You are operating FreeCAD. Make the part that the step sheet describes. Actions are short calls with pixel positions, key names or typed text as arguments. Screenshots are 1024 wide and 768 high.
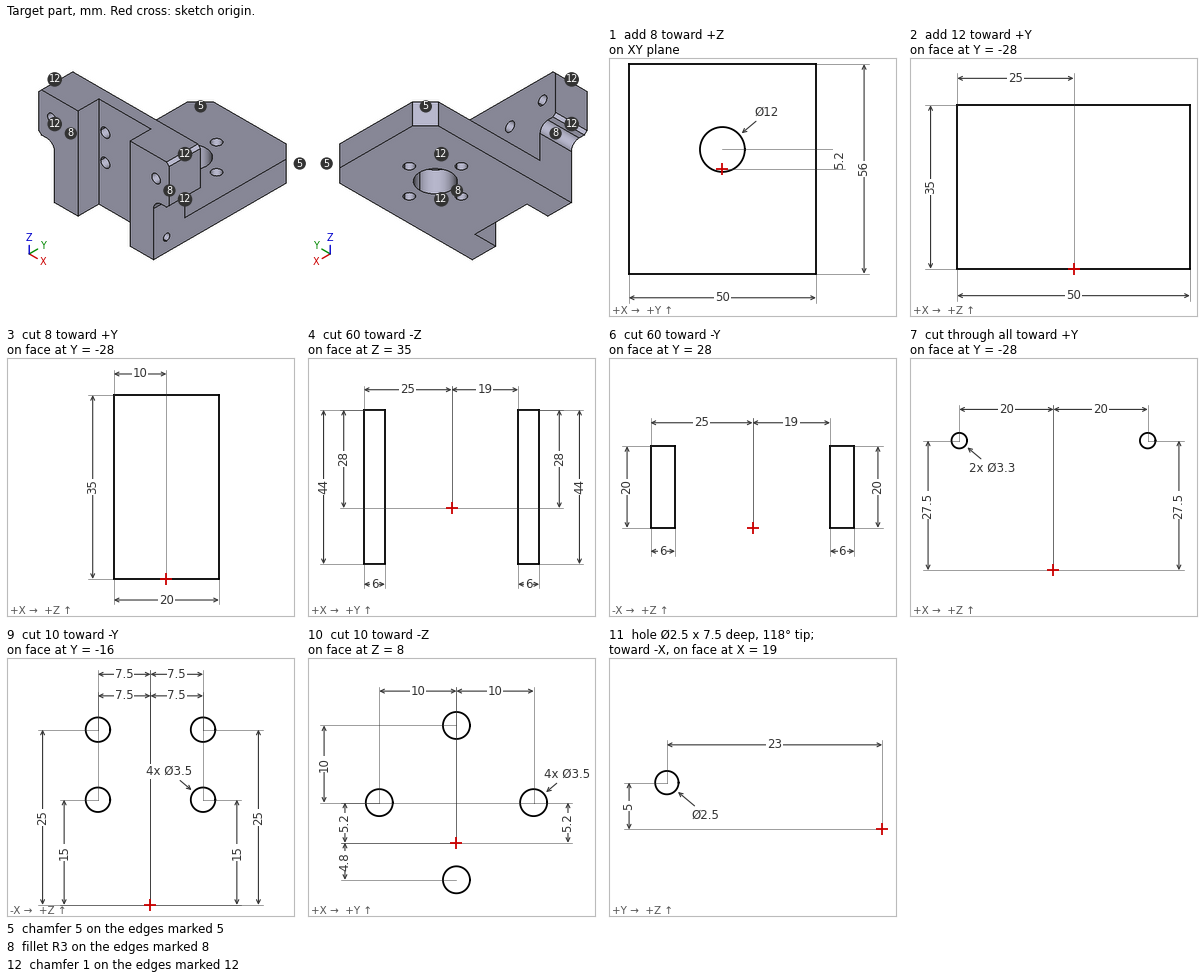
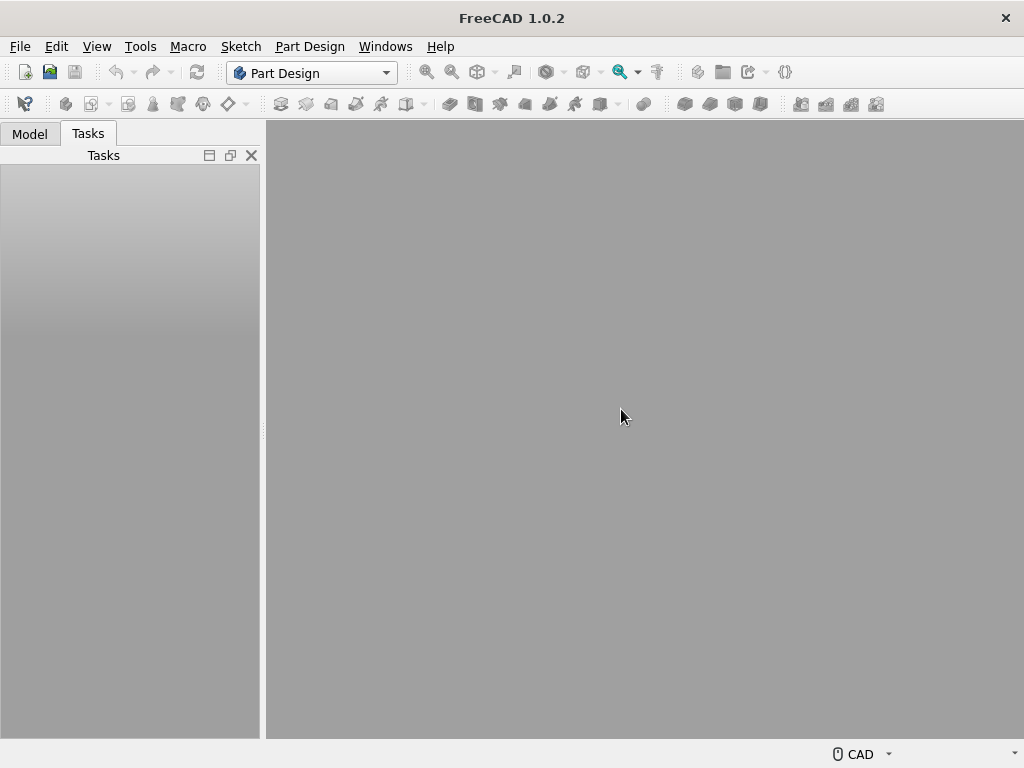
click(25, 72)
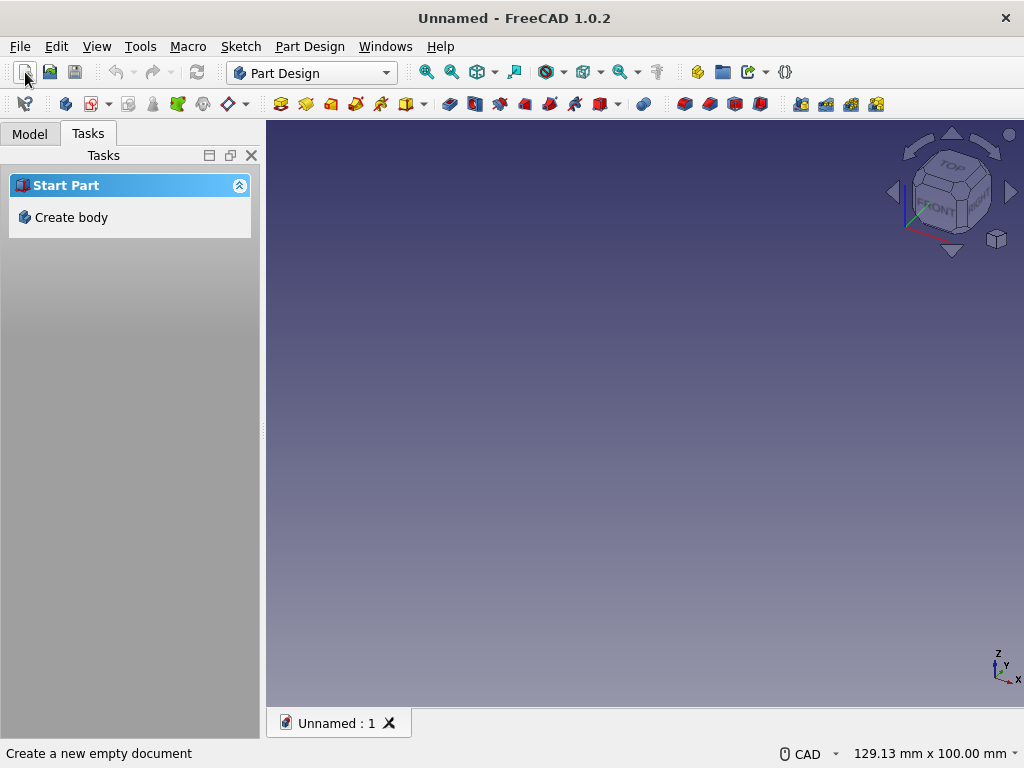
click(90, 104)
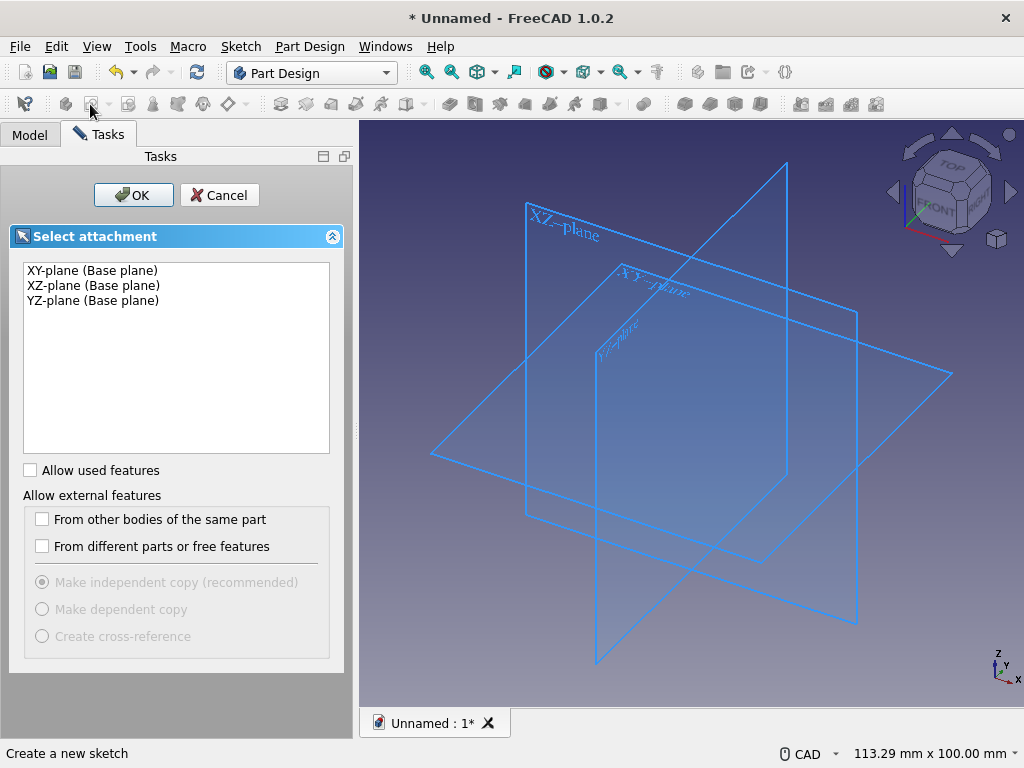
click(84, 270)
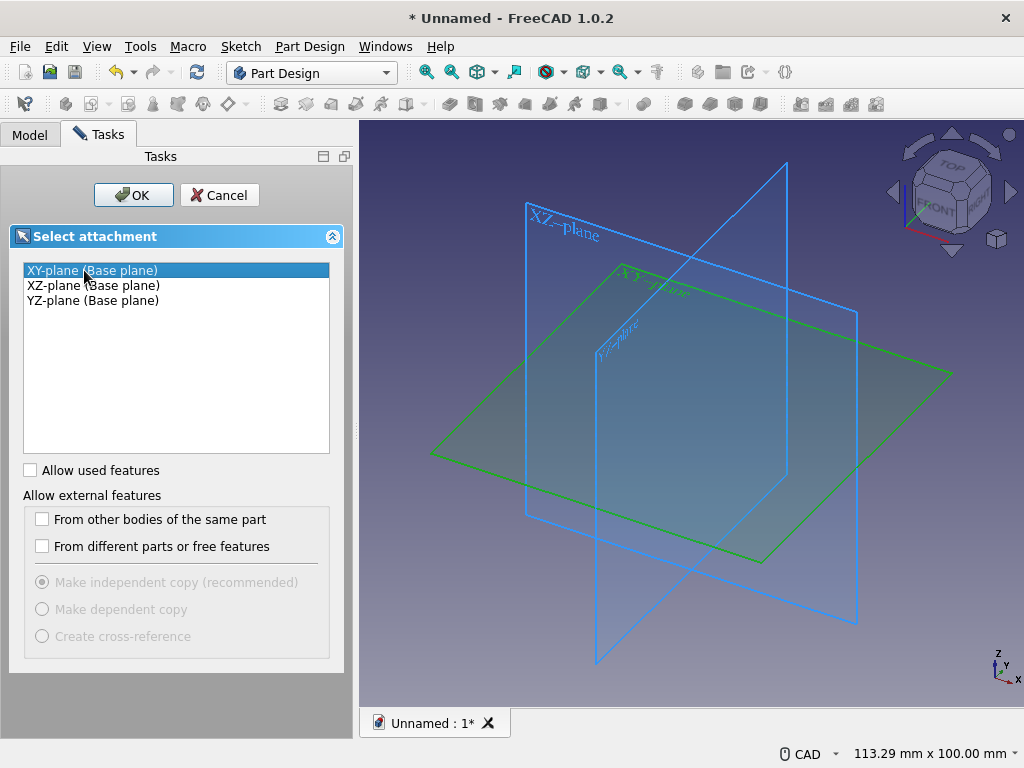
click(134, 195)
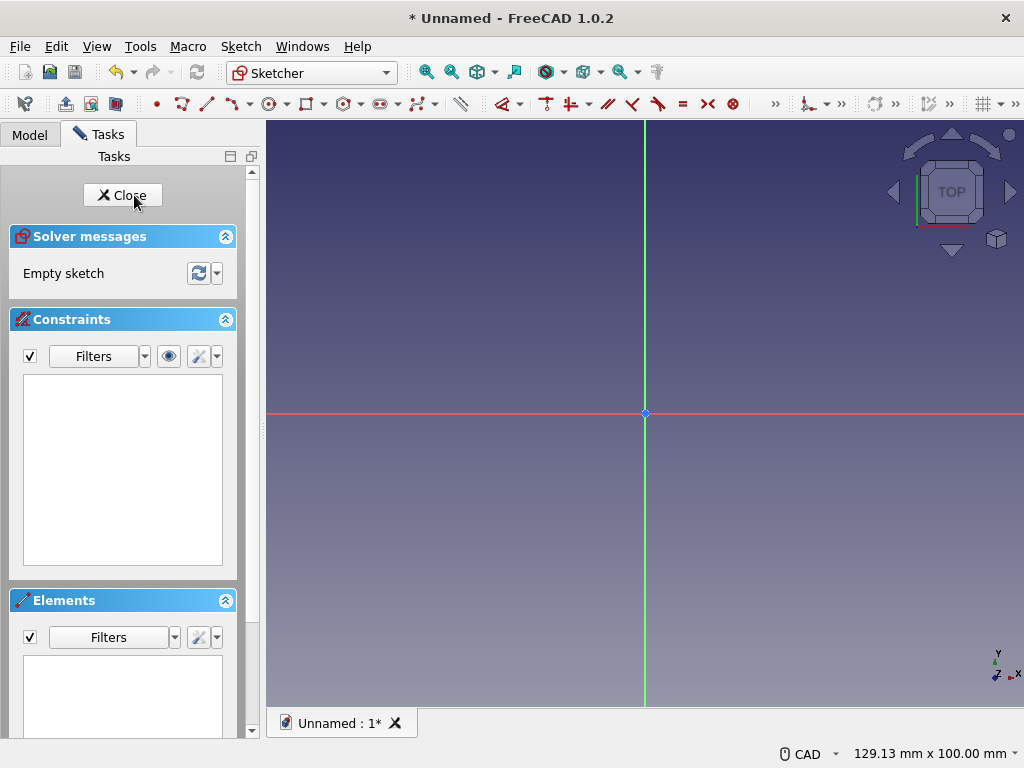
key(g)
key(v)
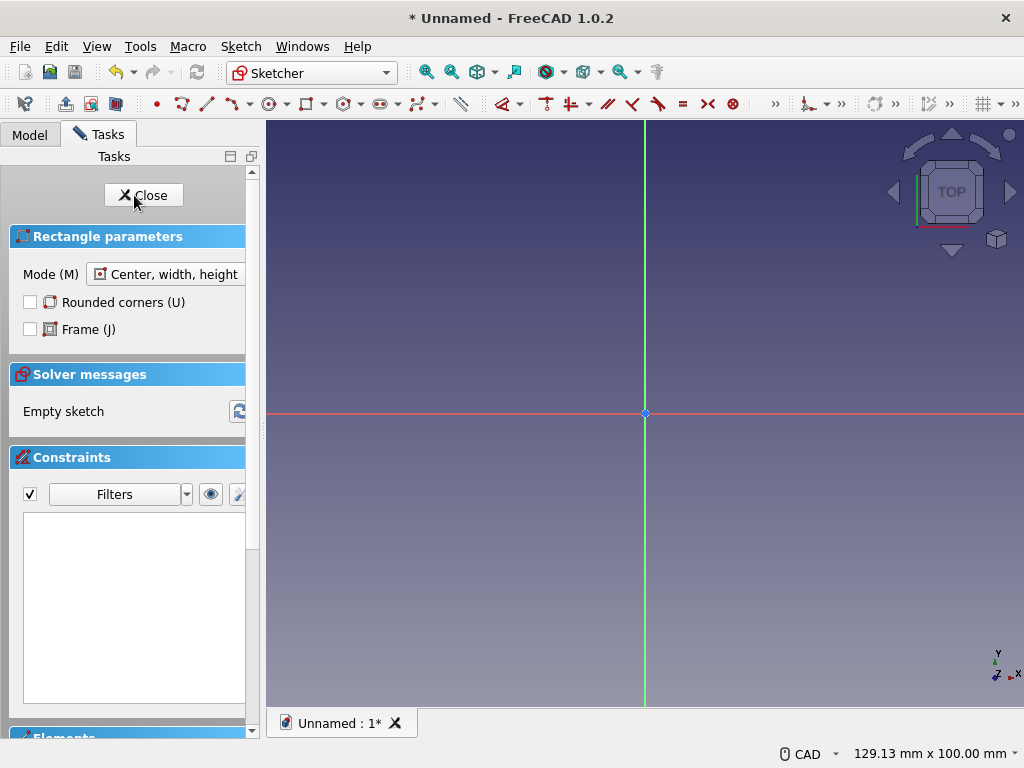
click(645, 414)
move(792, 249)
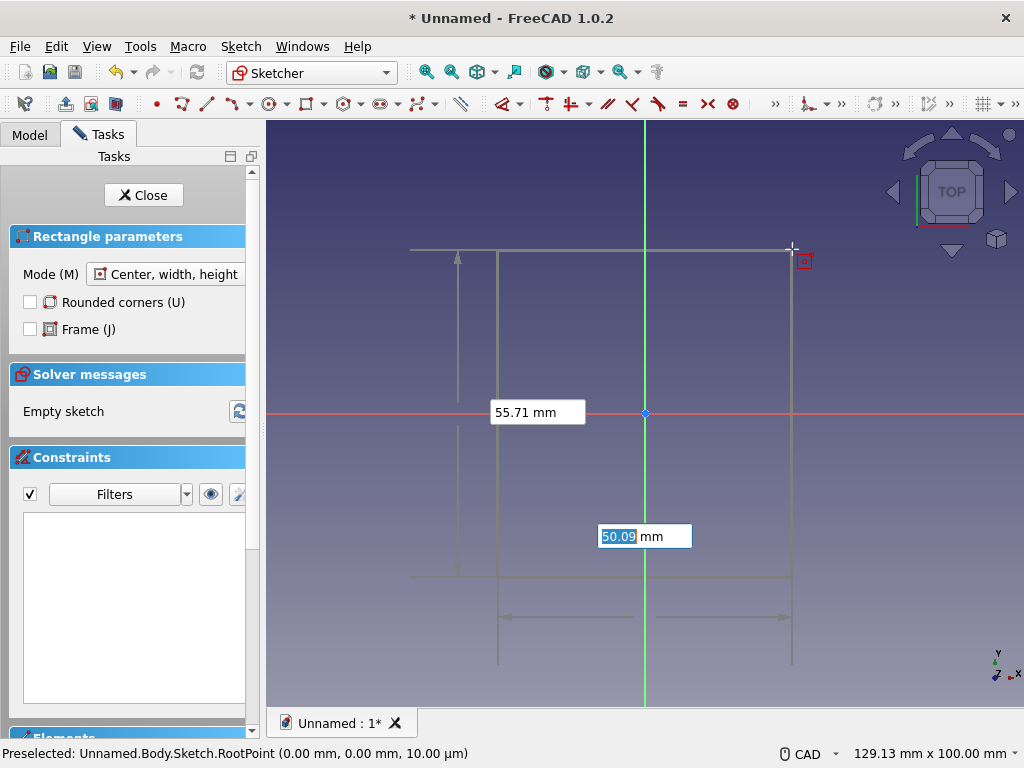
text(50)
key(Tab)
text(56)
key(Return)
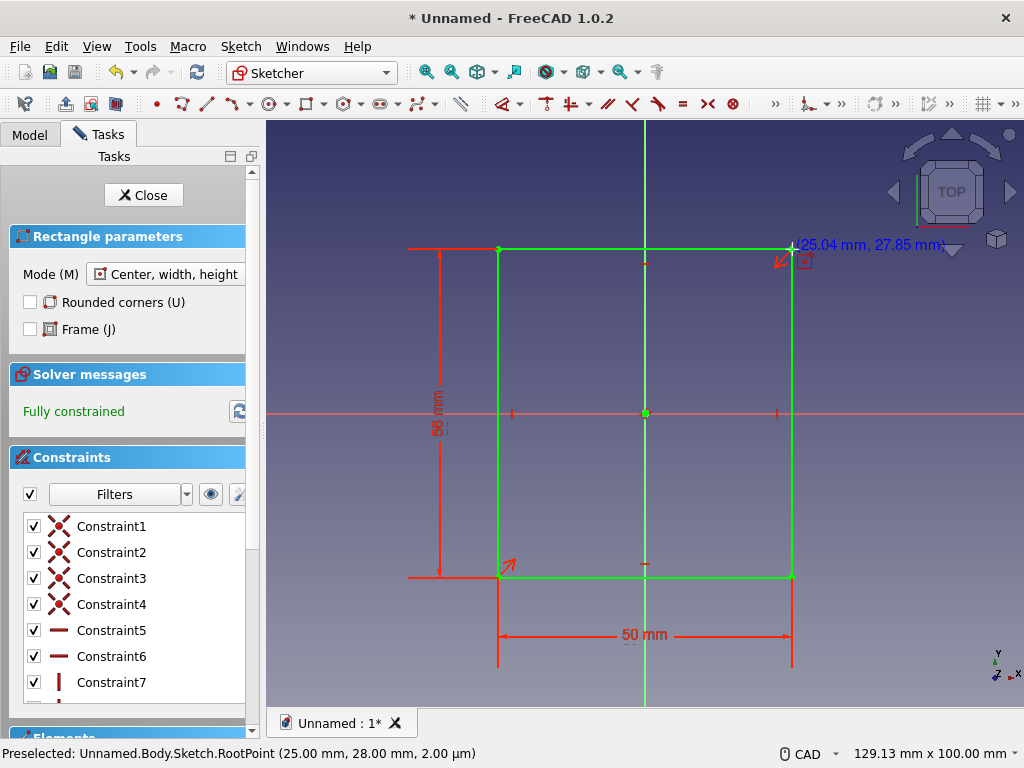
click(268, 104)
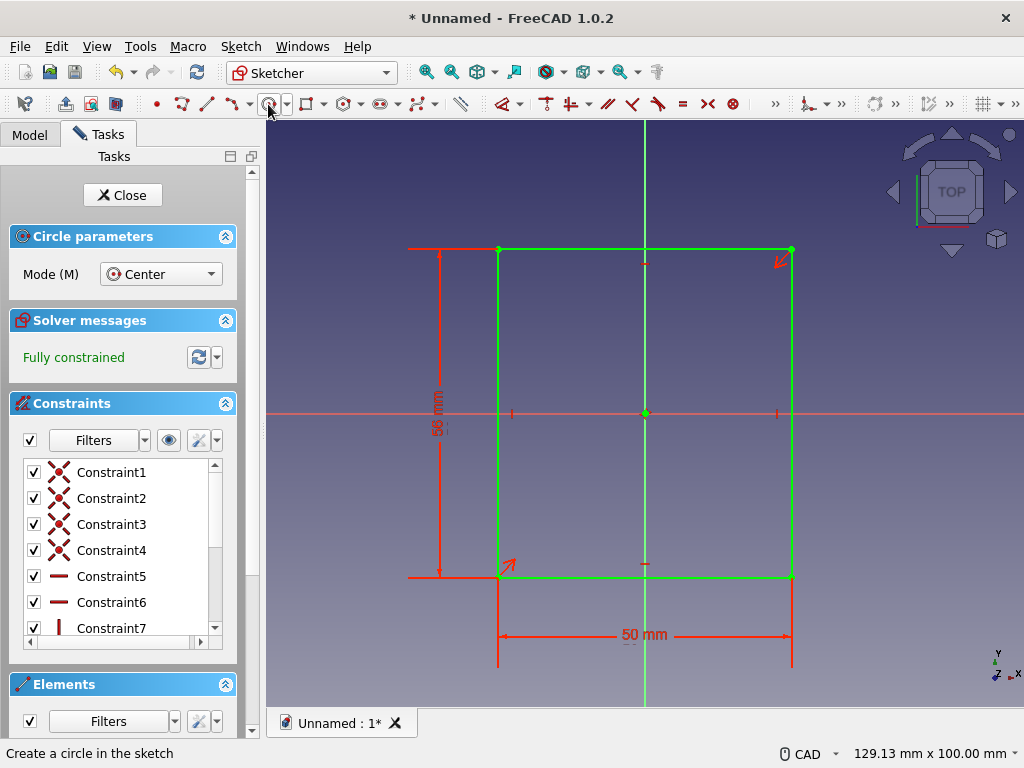
click(645, 383)
move(670, 358)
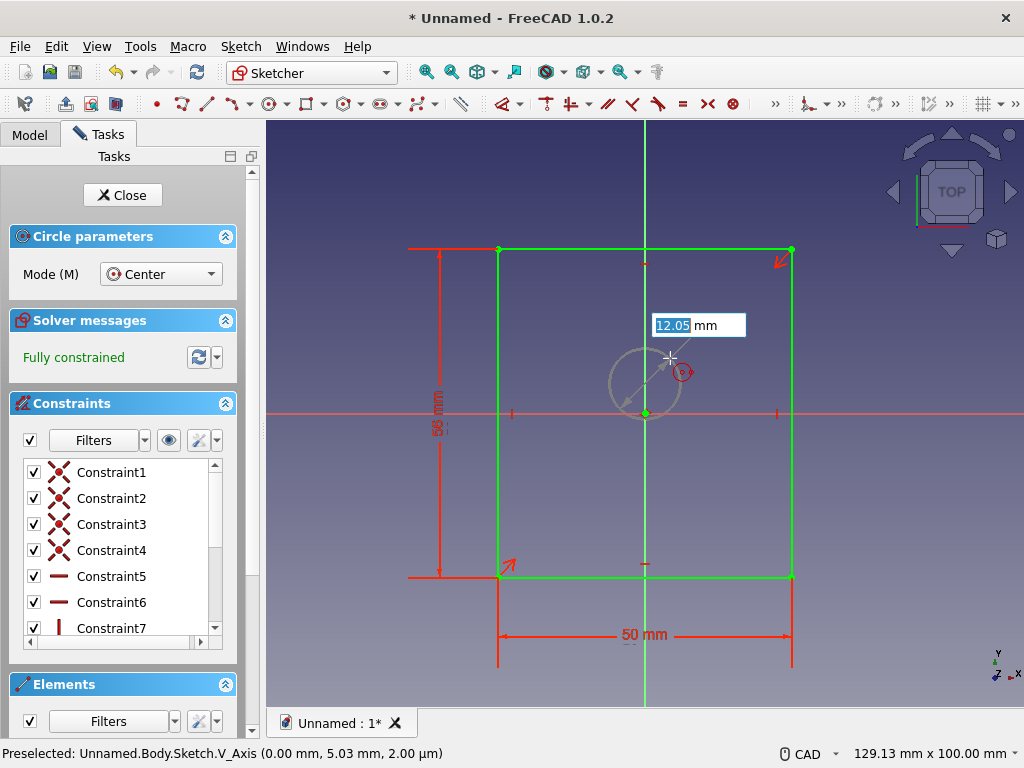
text(12)
key(Return)
key(Escape)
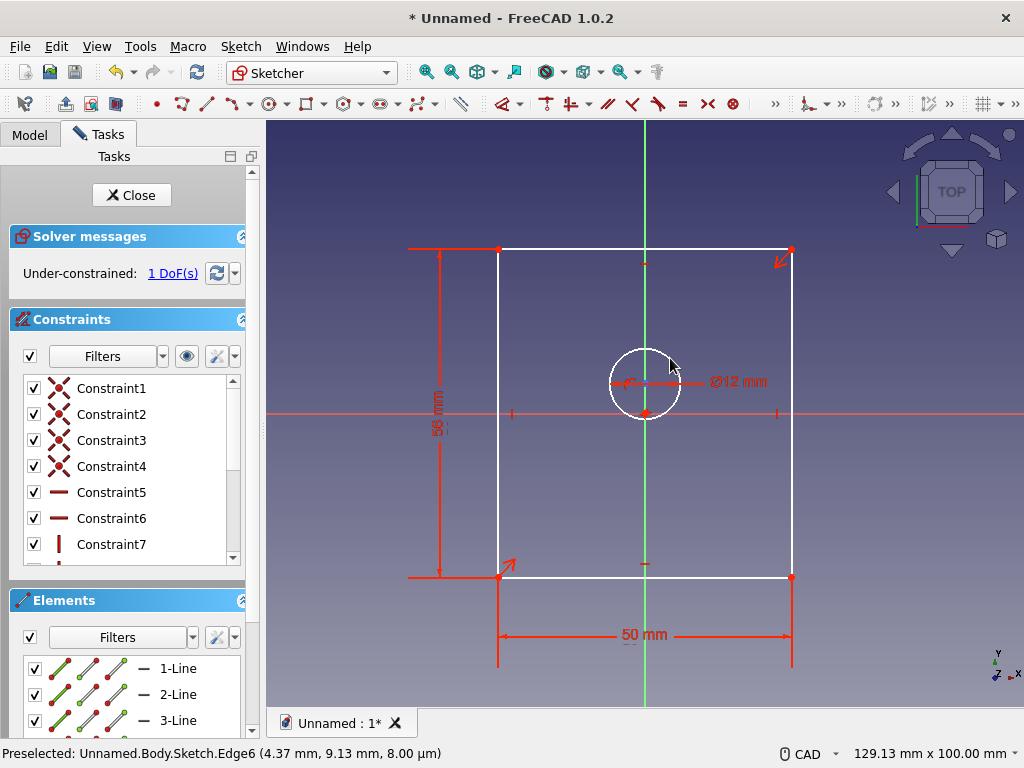
click(502, 104)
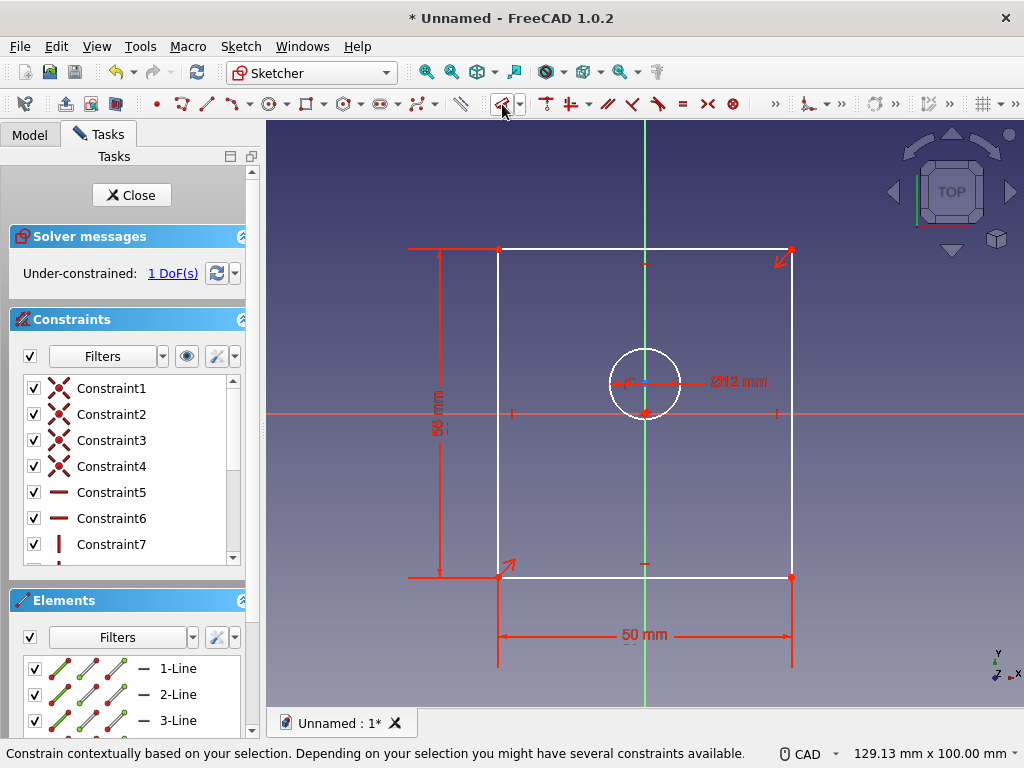
scroll(645, 384, up, 2)